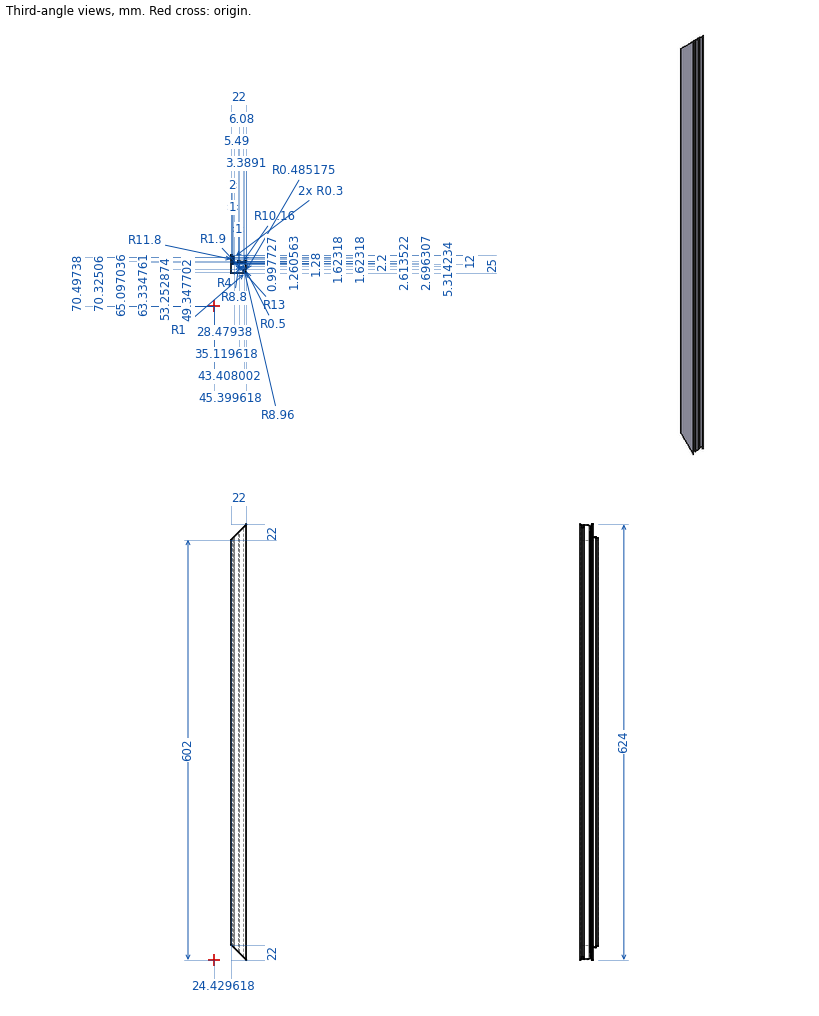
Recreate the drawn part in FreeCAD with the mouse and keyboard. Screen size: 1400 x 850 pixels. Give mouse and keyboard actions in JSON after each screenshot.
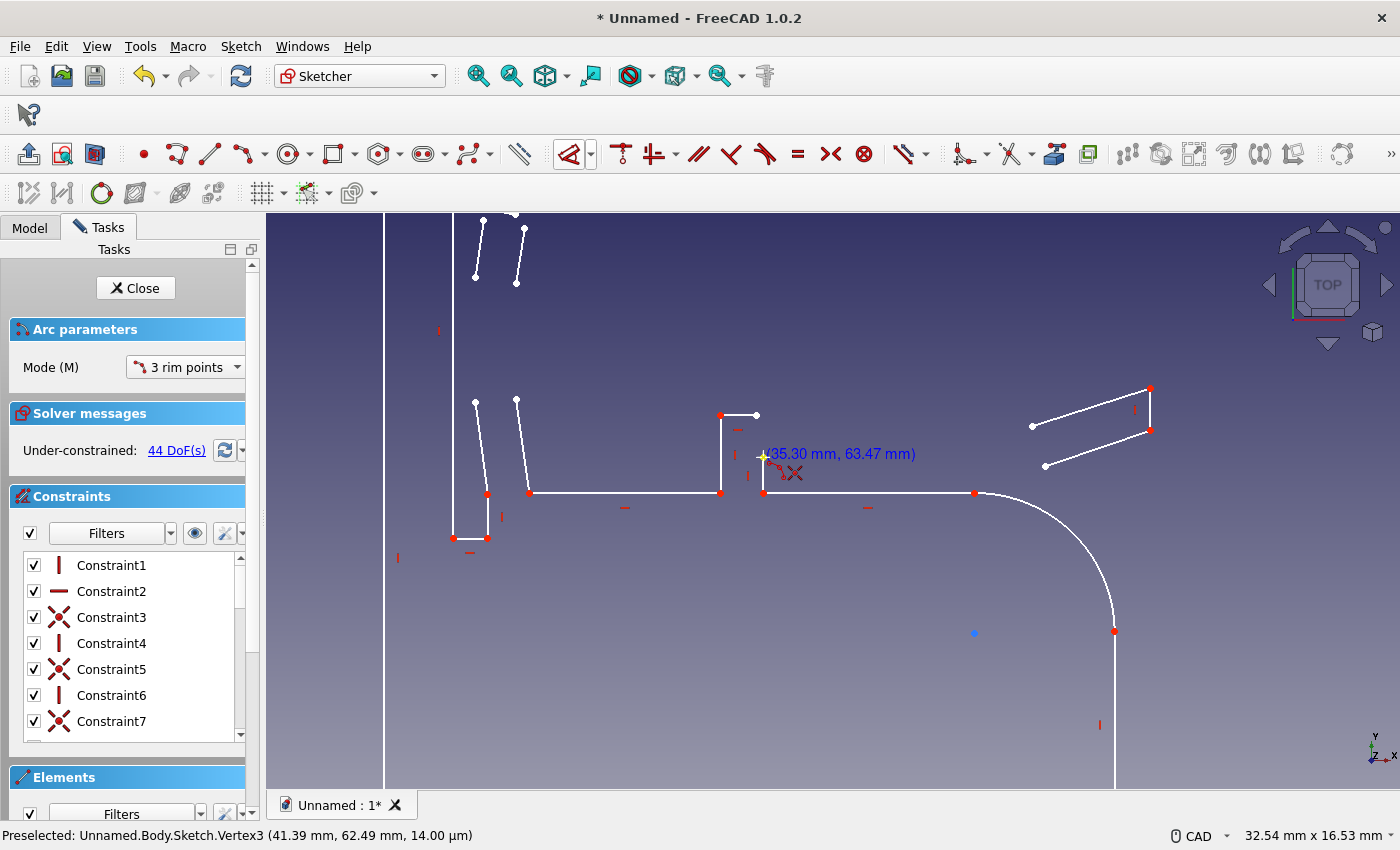
{"action": "left_click", "coordinate": [763, 457]}
{"action": "left_click", "coordinate": [840, 467]}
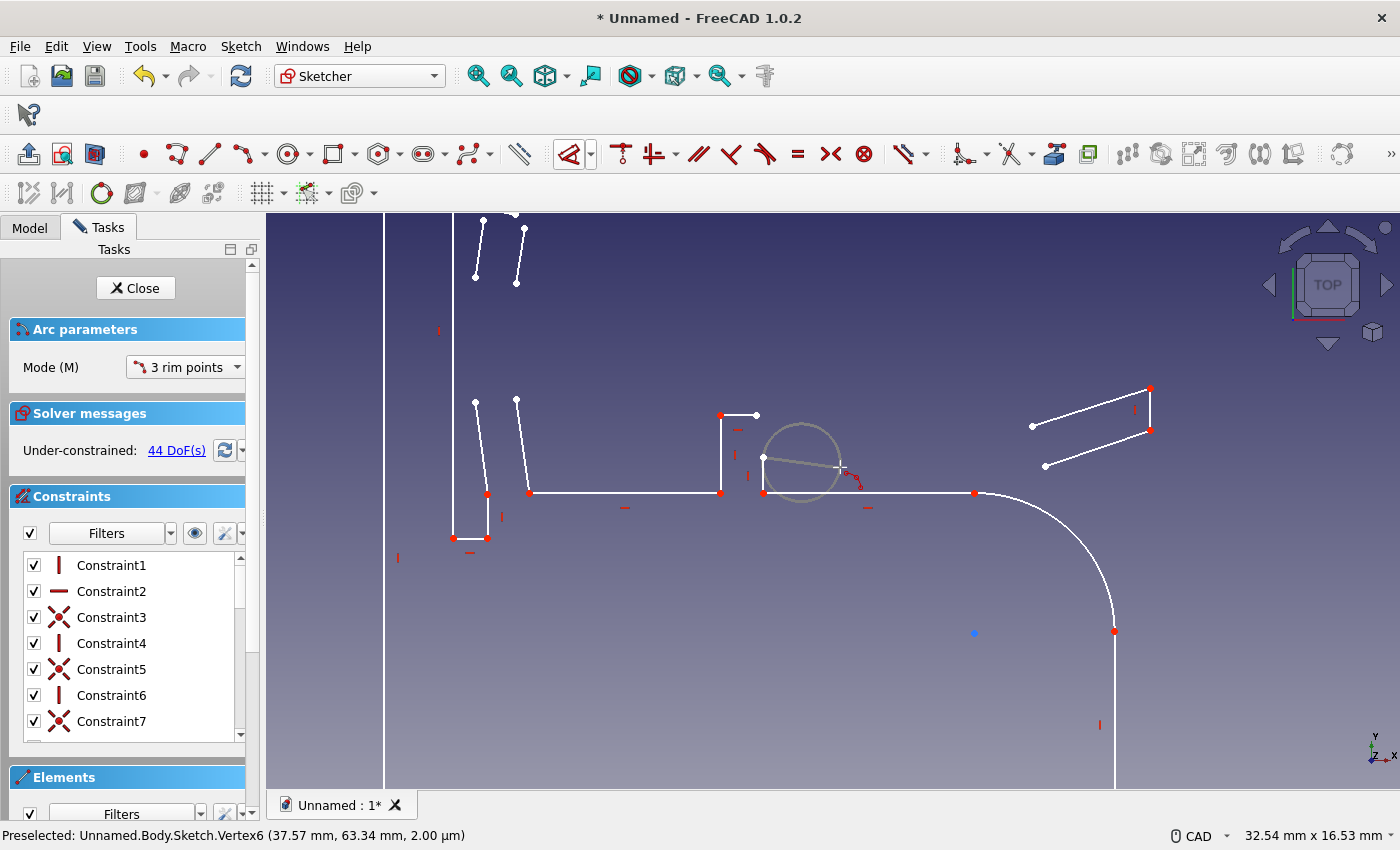
{"action": "scroll", "coordinate": [802, 459], "scroll_direction": "up", "scroll_amount": 10}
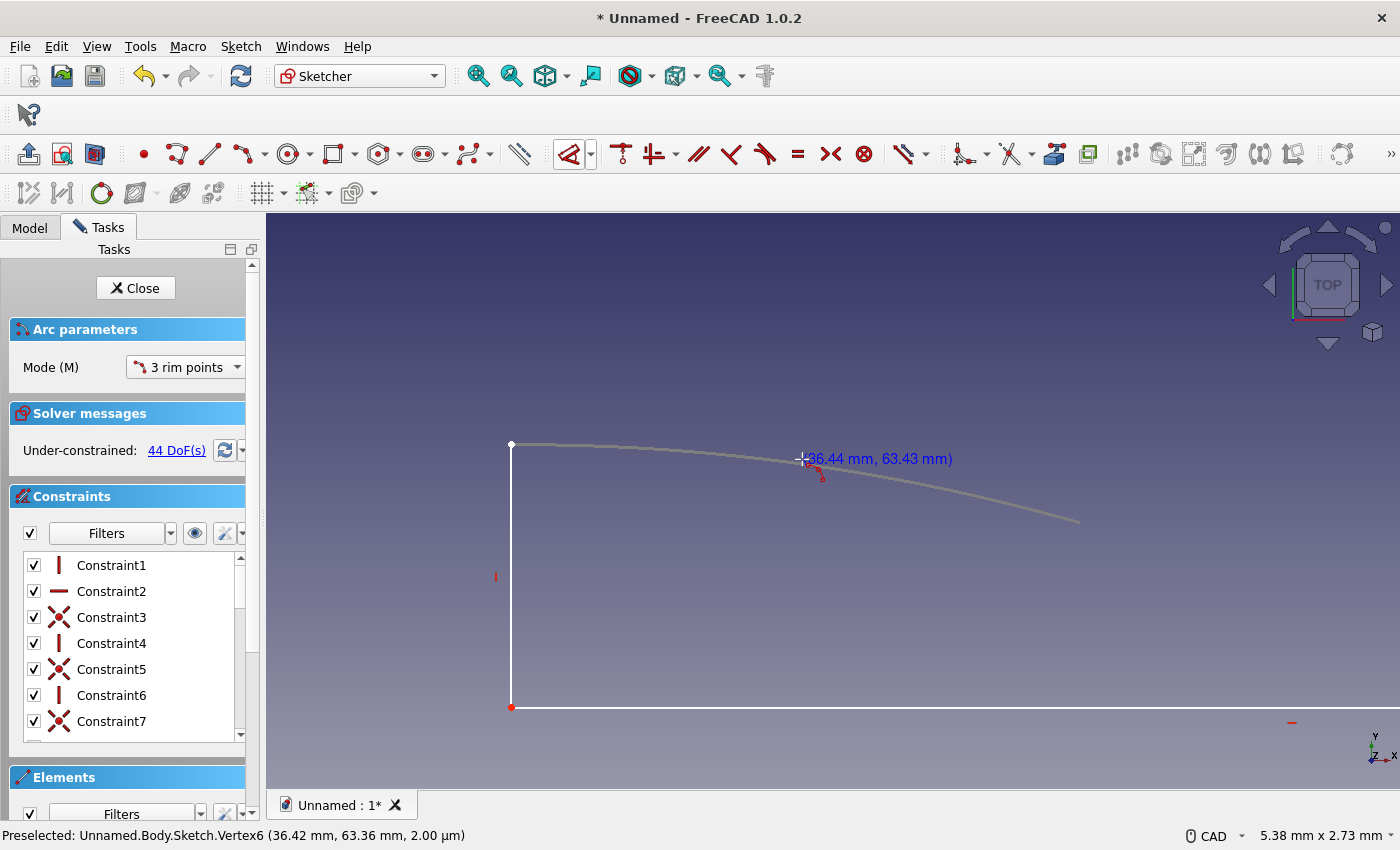
{"action": "left_click", "coordinate": [798, 455]}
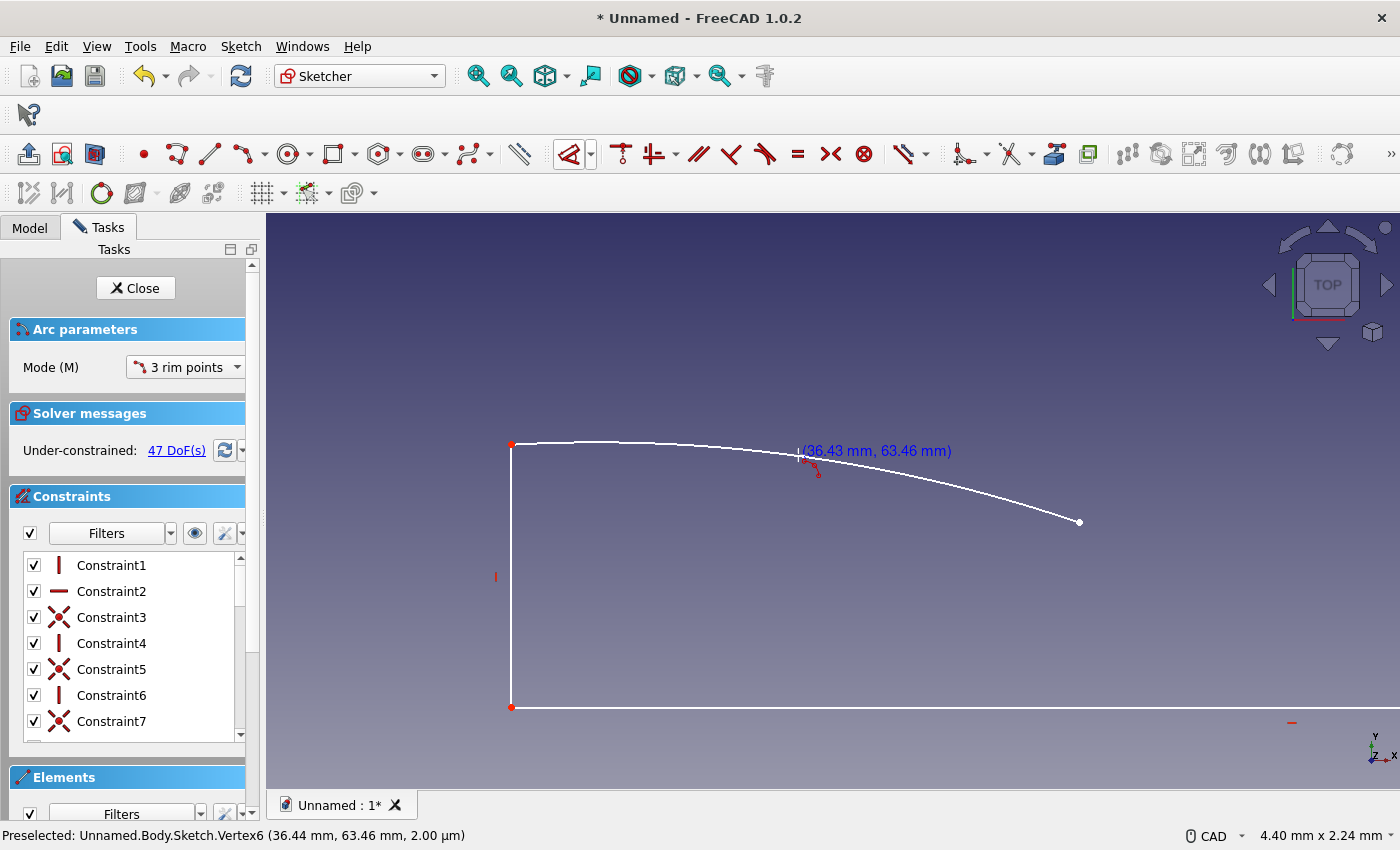
{"action": "scroll", "coordinate": [779, 458], "scroll_direction": "down", "scroll_amount": 14}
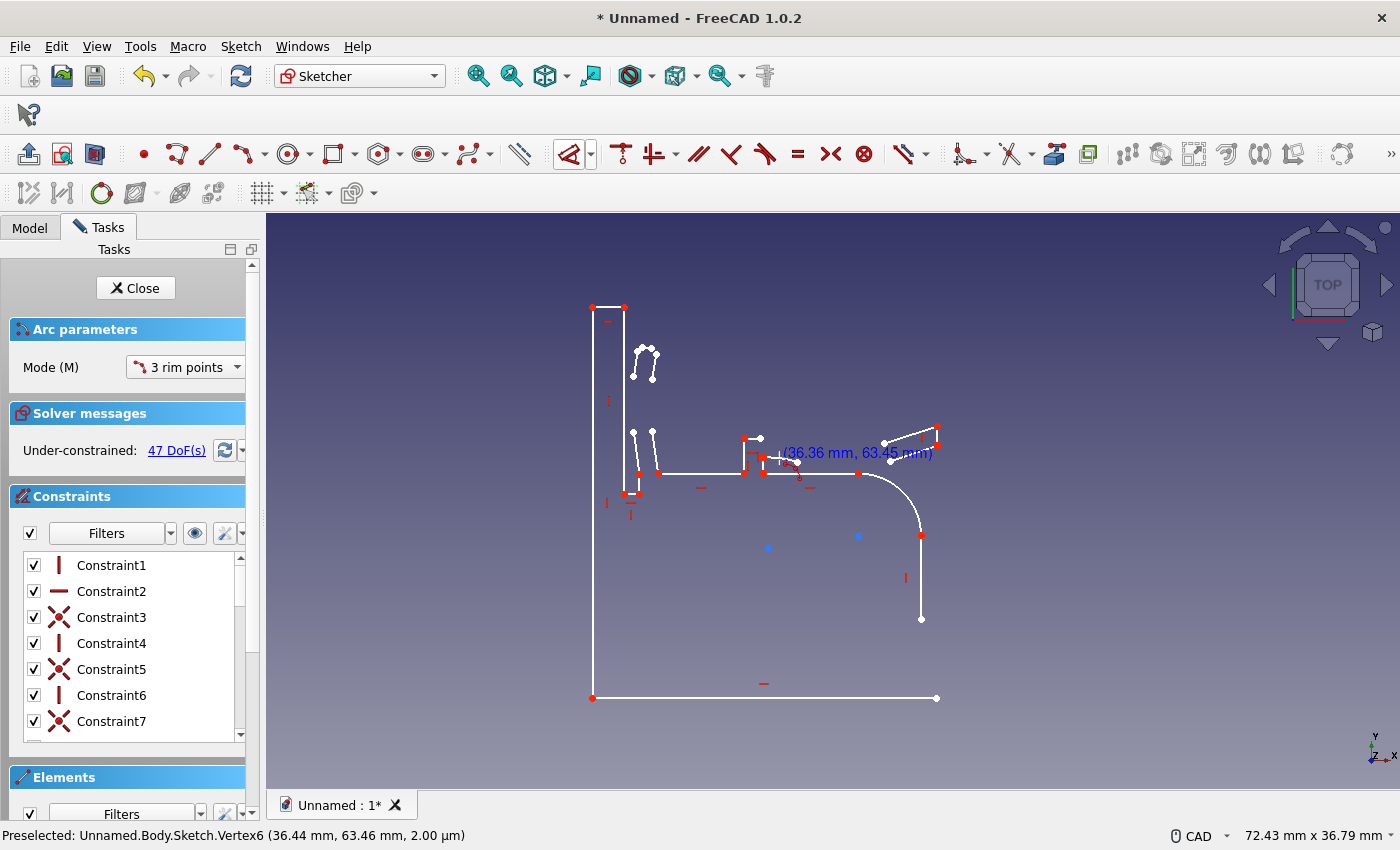
{"action": "scroll", "coordinate": [798, 462], "scroll_direction": "up", "scroll_amount": 3}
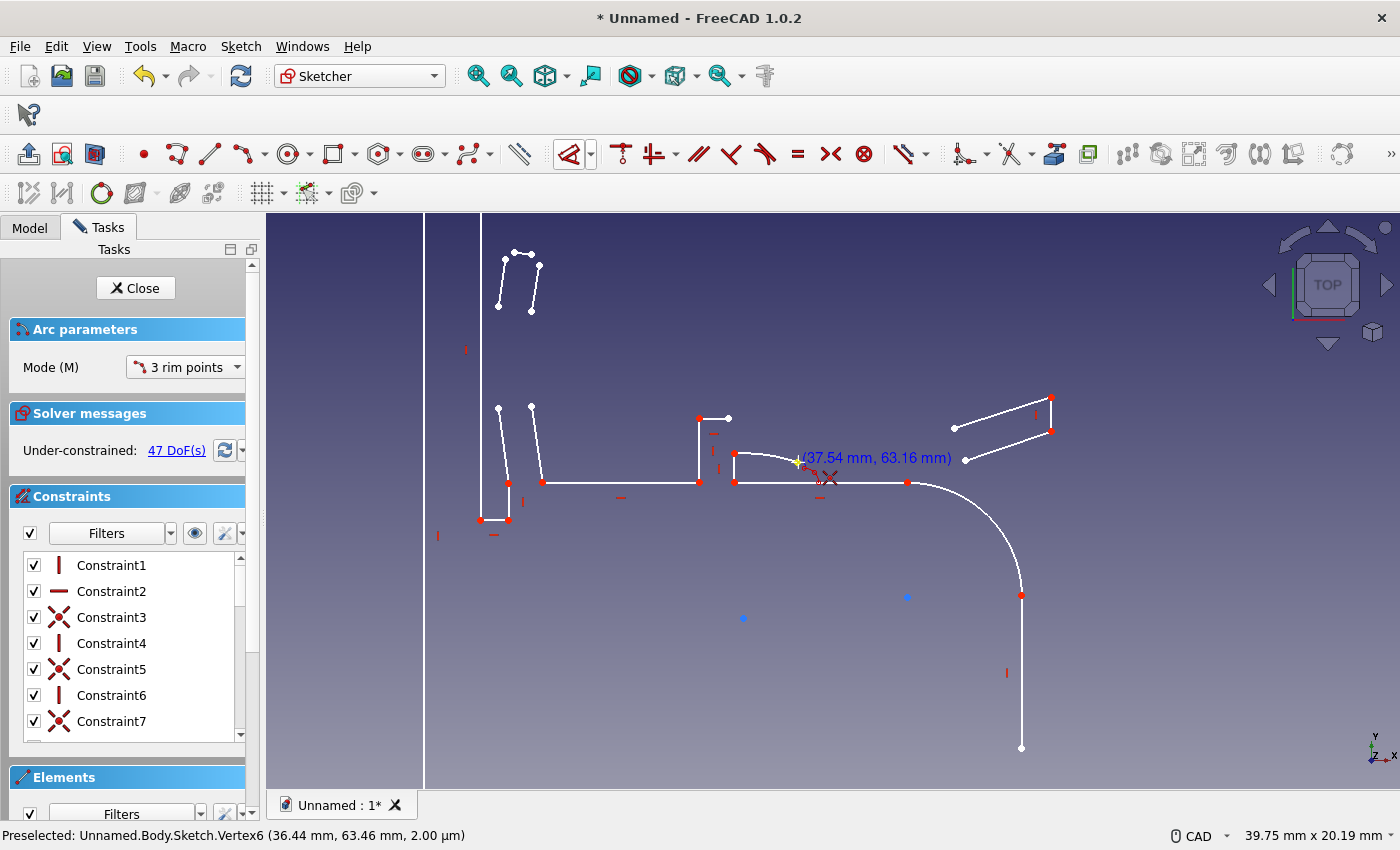
{"action": "left_click", "coordinate": [797, 462]}
{"action": "left_click", "coordinate": [966, 461]}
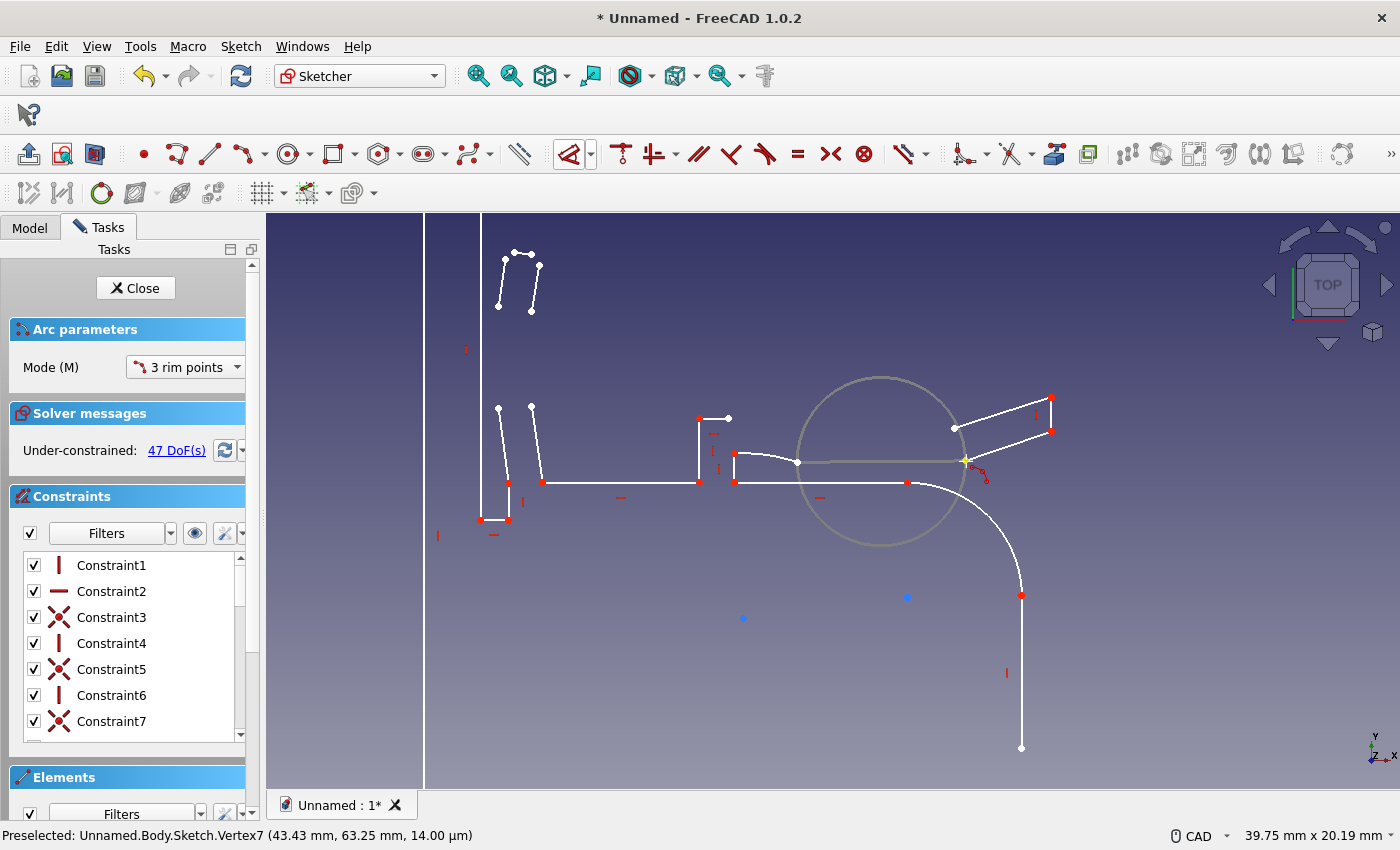
{"action": "scroll", "coordinate": [915, 470], "scroll_direction": "up", "scroll_amount": 3}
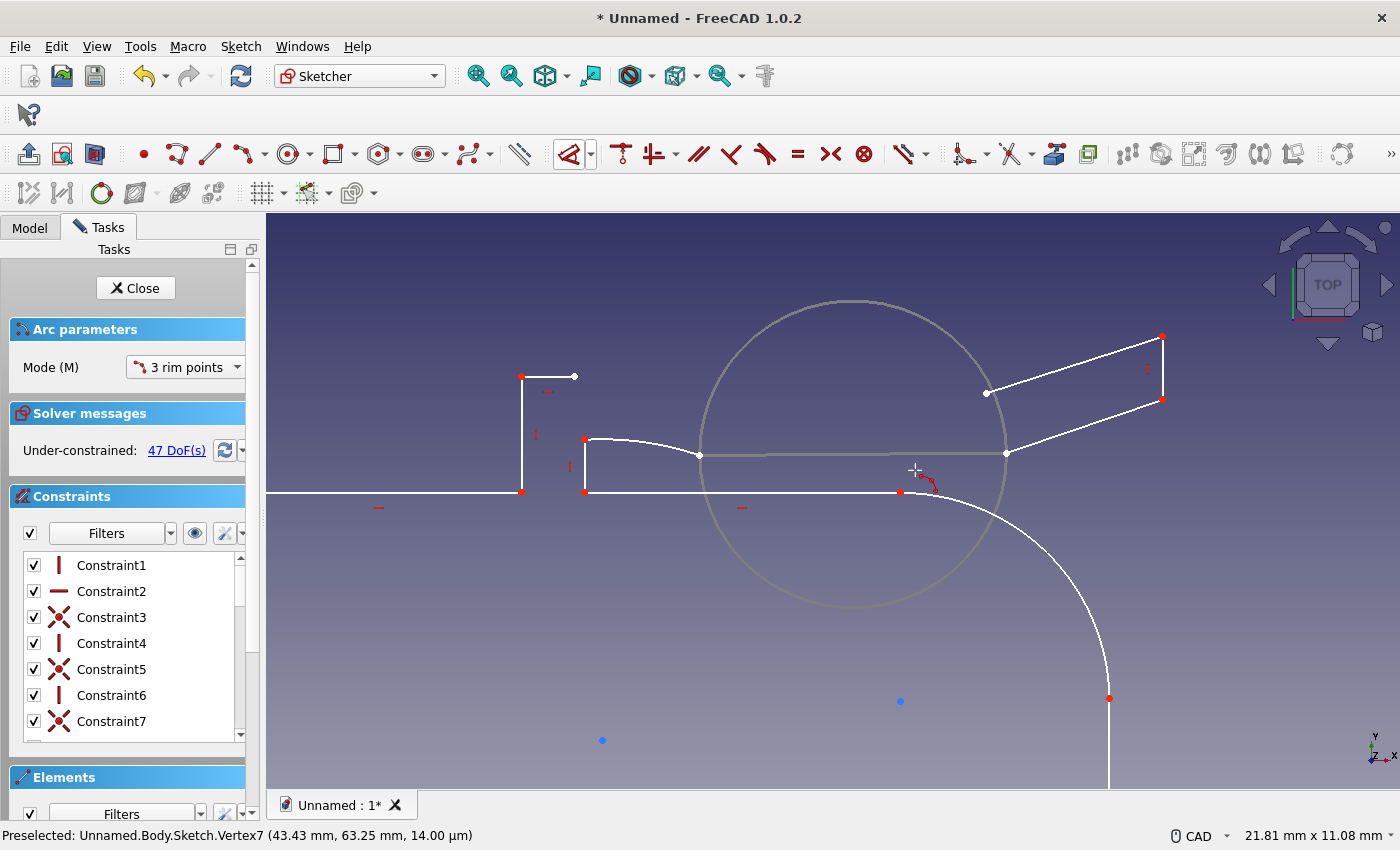
{"action": "left_click", "coordinate": [915, 469]}